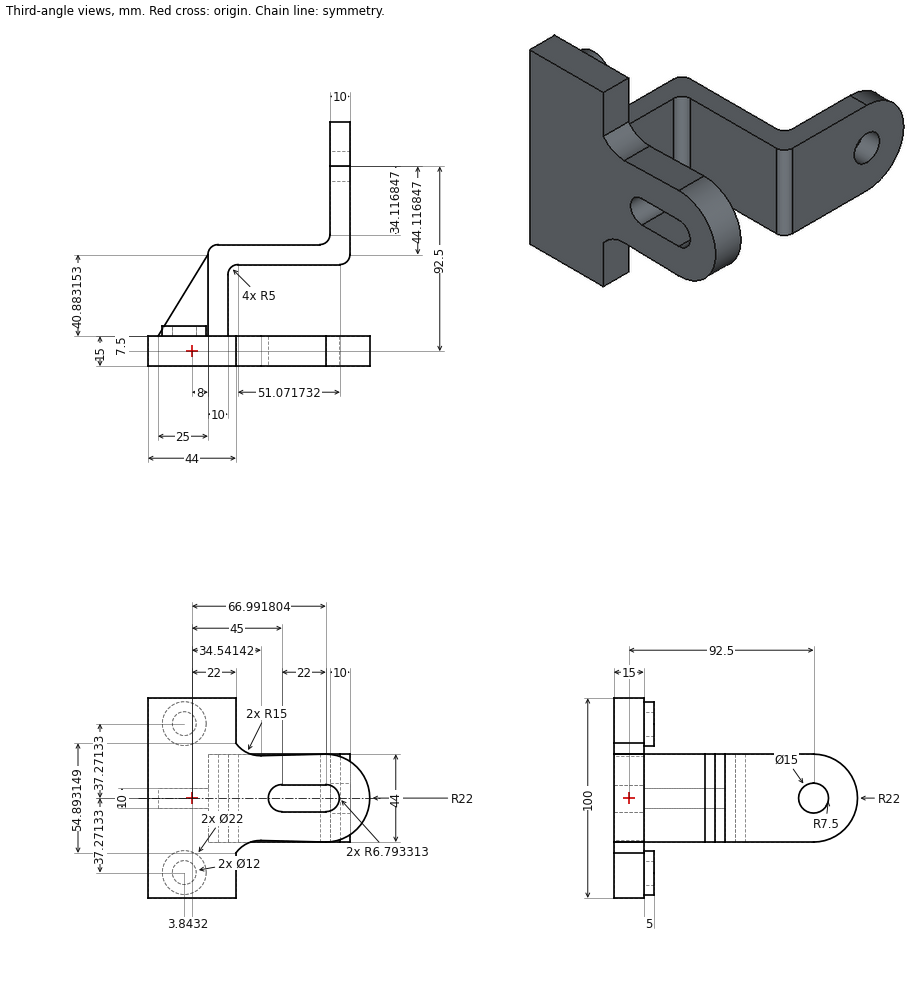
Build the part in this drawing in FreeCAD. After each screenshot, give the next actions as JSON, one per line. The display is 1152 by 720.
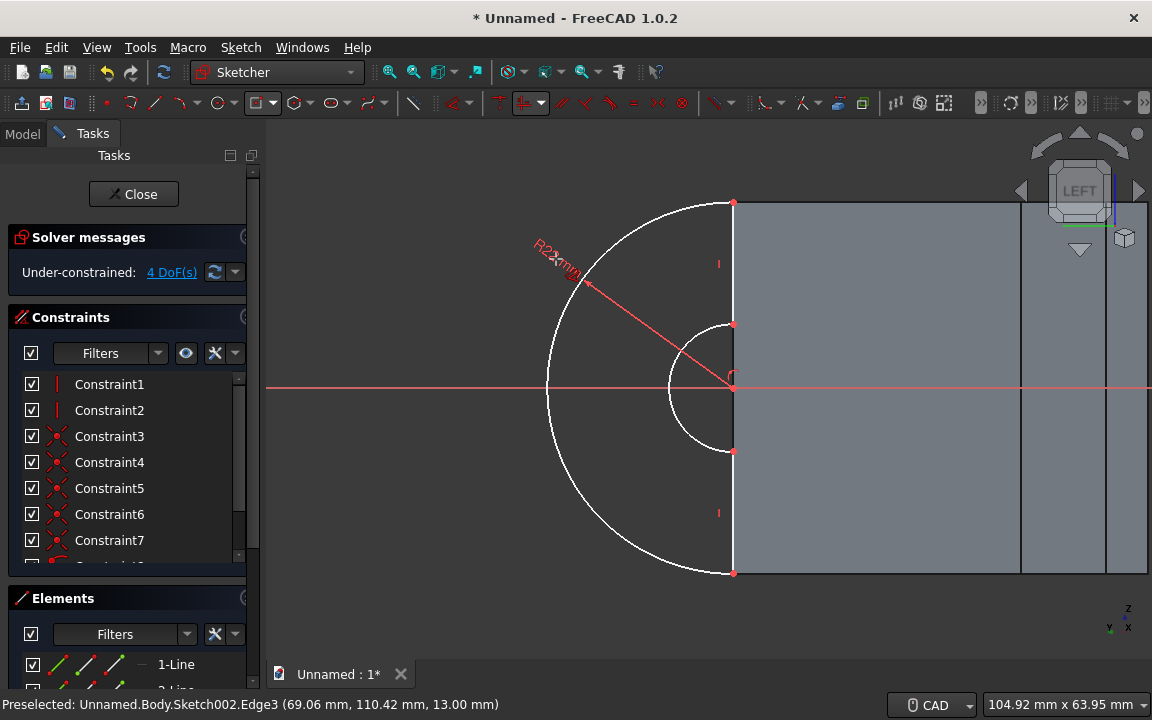
{"action": "left_click", "coordinate": [681, 351]}
{"action": "left_click", "coordinate": [655, 332]}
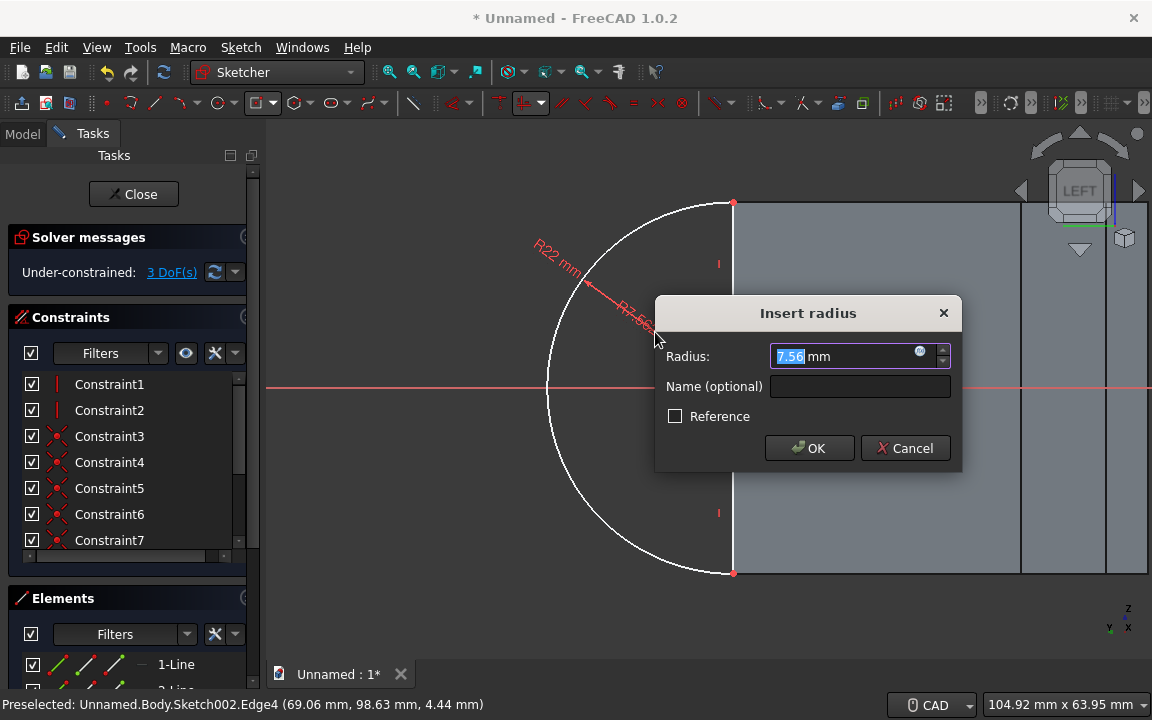
{"action": "type", "text": "7.5"}
{"action": "key", "text": "Return"}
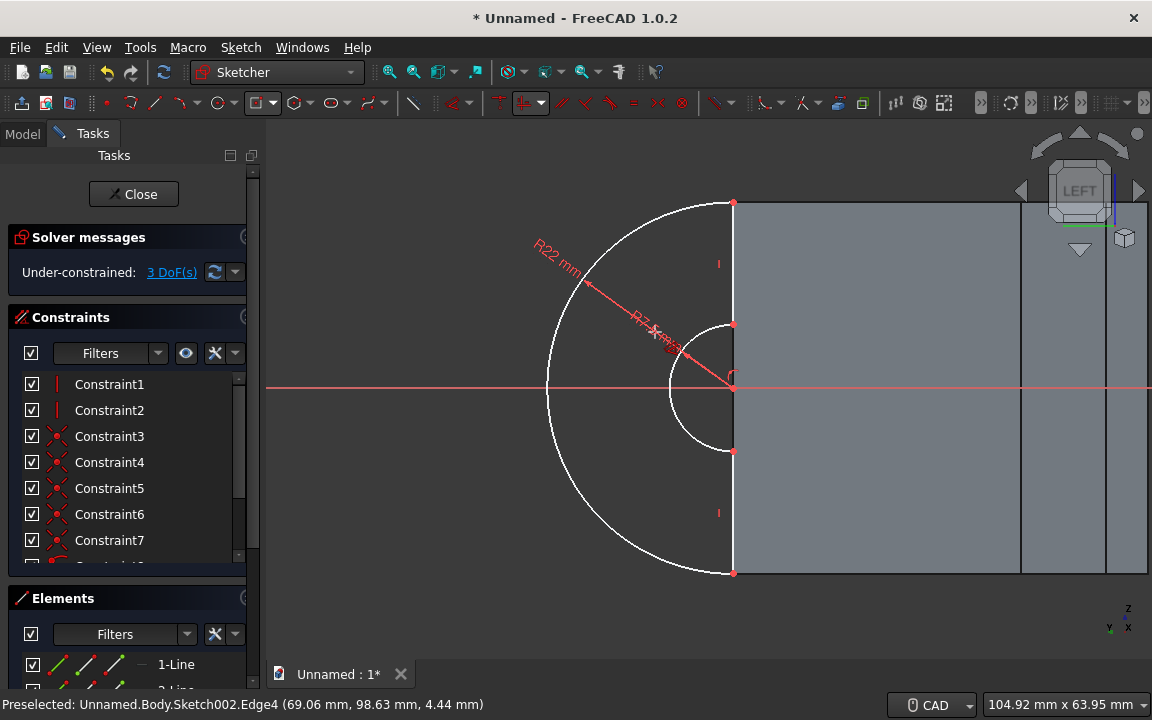
{"action": "left_click", "coordinate": [733, 325]}
{"action": "left_click", "coordinate": [860, 291]}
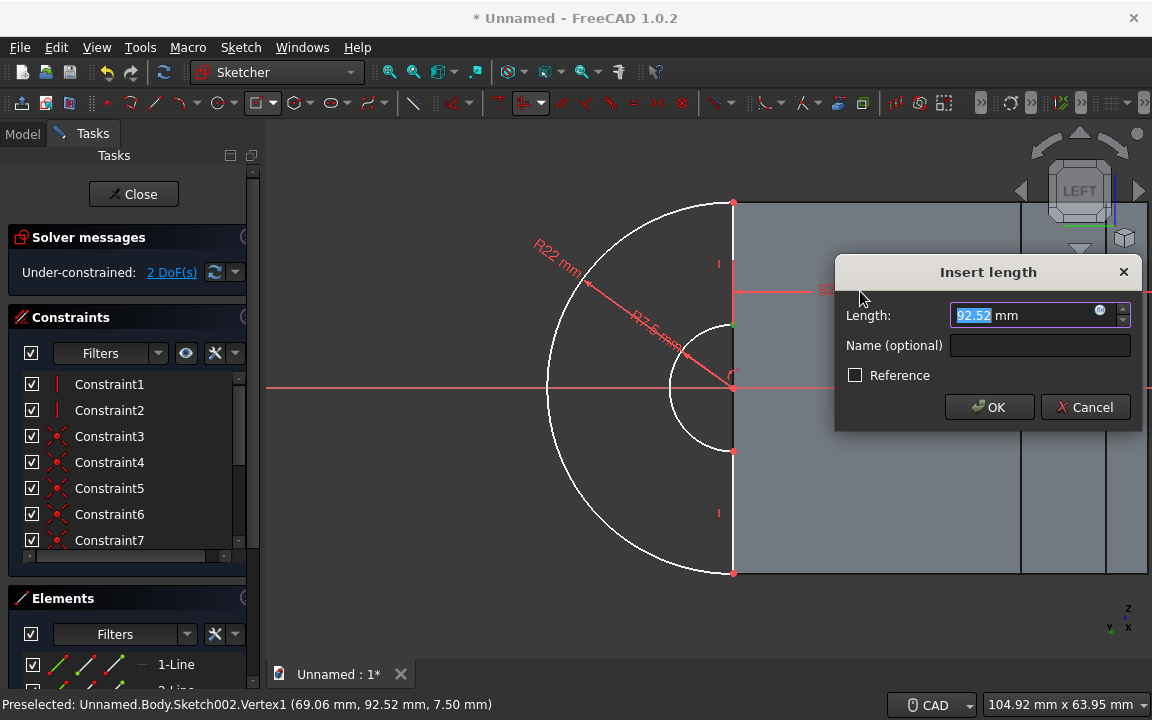
{"action": "type", "text": "92.5"}
{"action": "key", "text": "Return"}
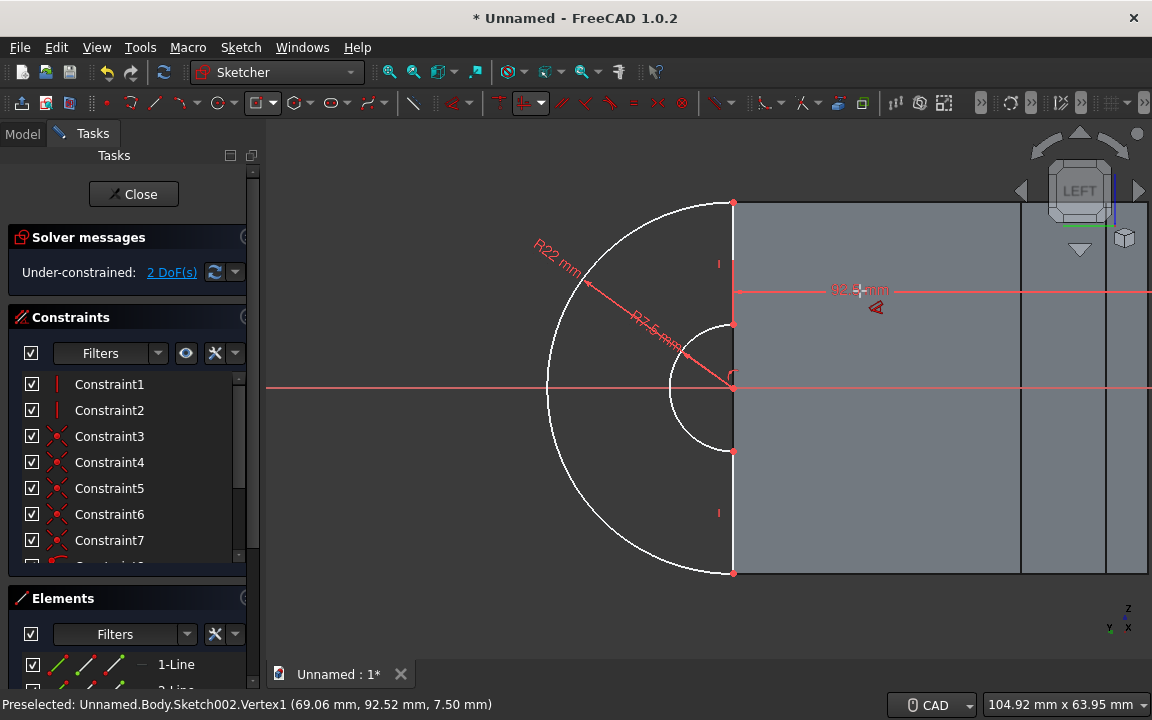
{"action": "left_click", "coordinate": [733, 574]}
{"action": "left_click", "coordinate": [860, 608]}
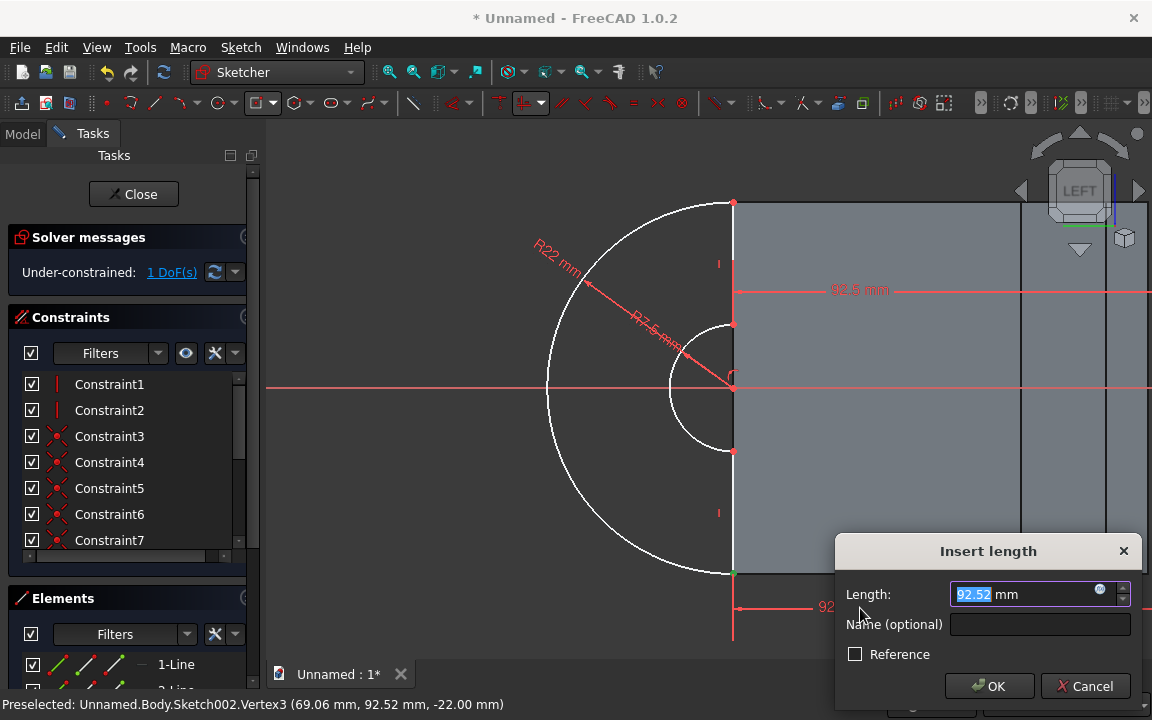
{"action": "type", "text": "92.5"}
{"action": "key", "text": "Return"}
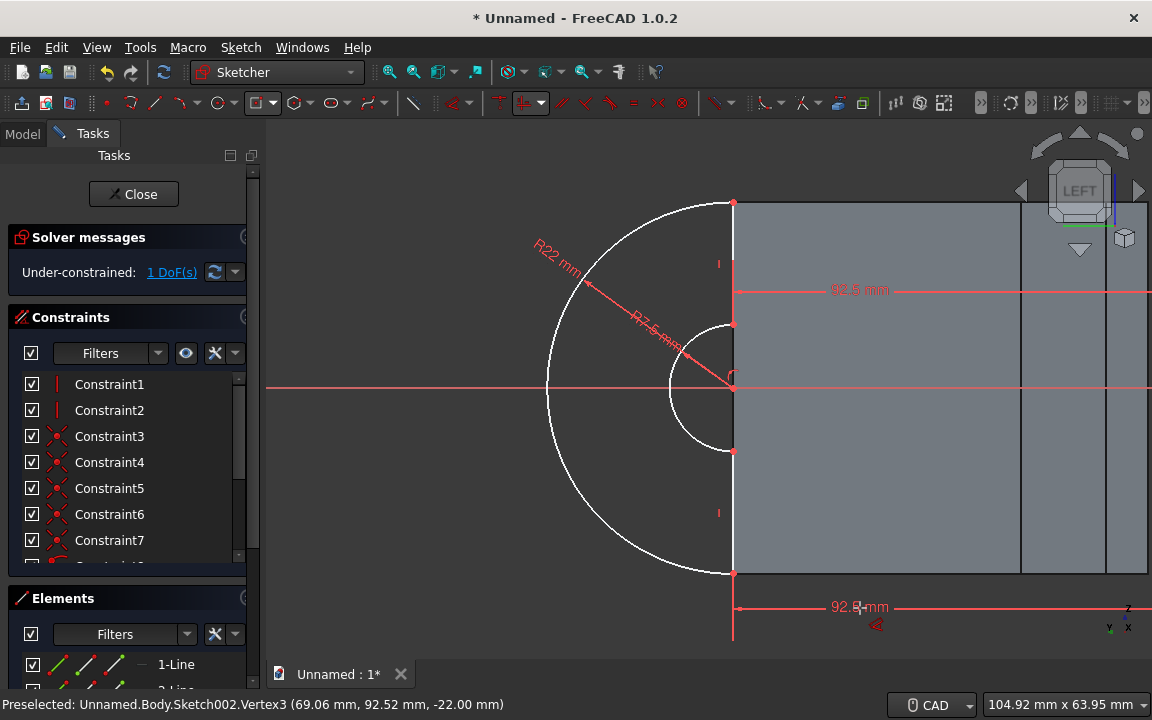
{"action": "left_click", "coordinate": [733, 388]}
{"action": "left_click", "coordinate": [860, 422]}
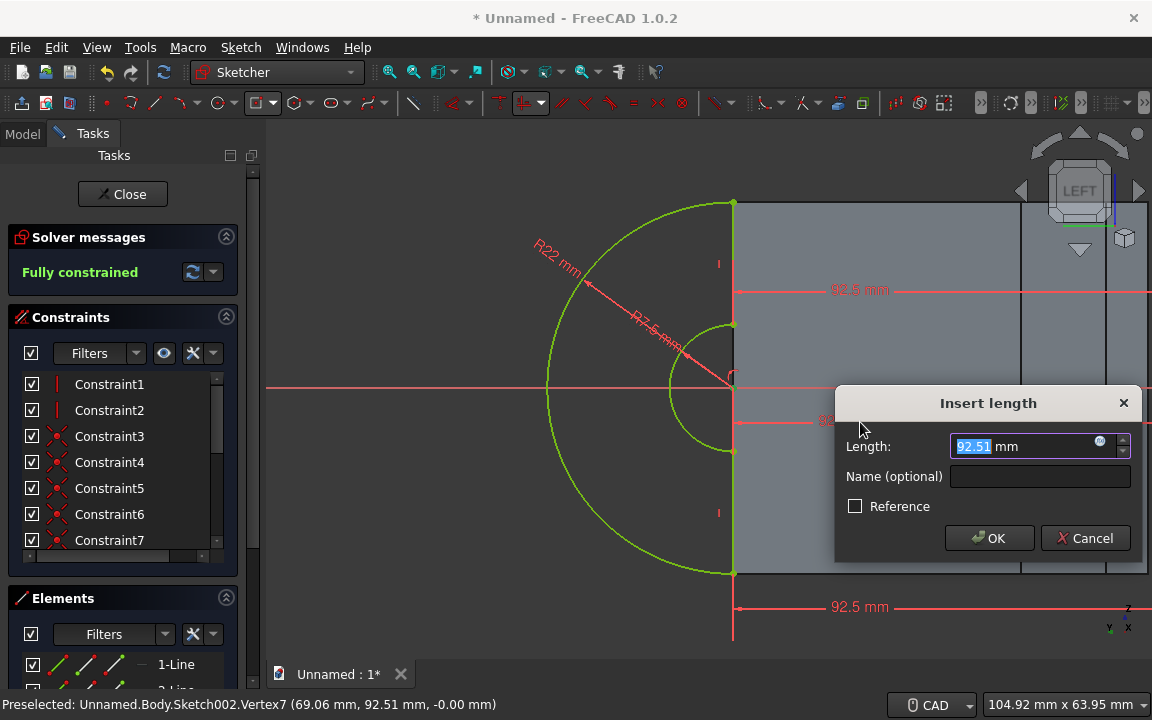
{"action": "type", "text": "92.5"}
{"action": "key", "text": "Return"}
{"action": "key", "text": "Escape"}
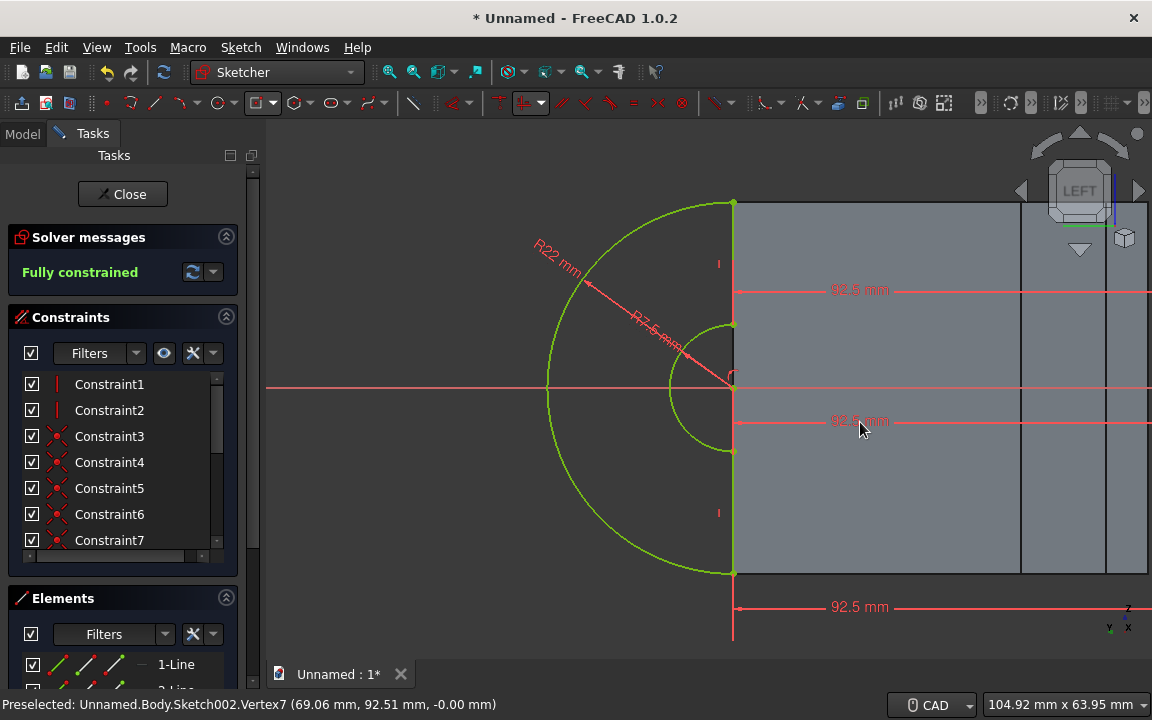
{"action": "left_click", "coordinate": [123, 194]}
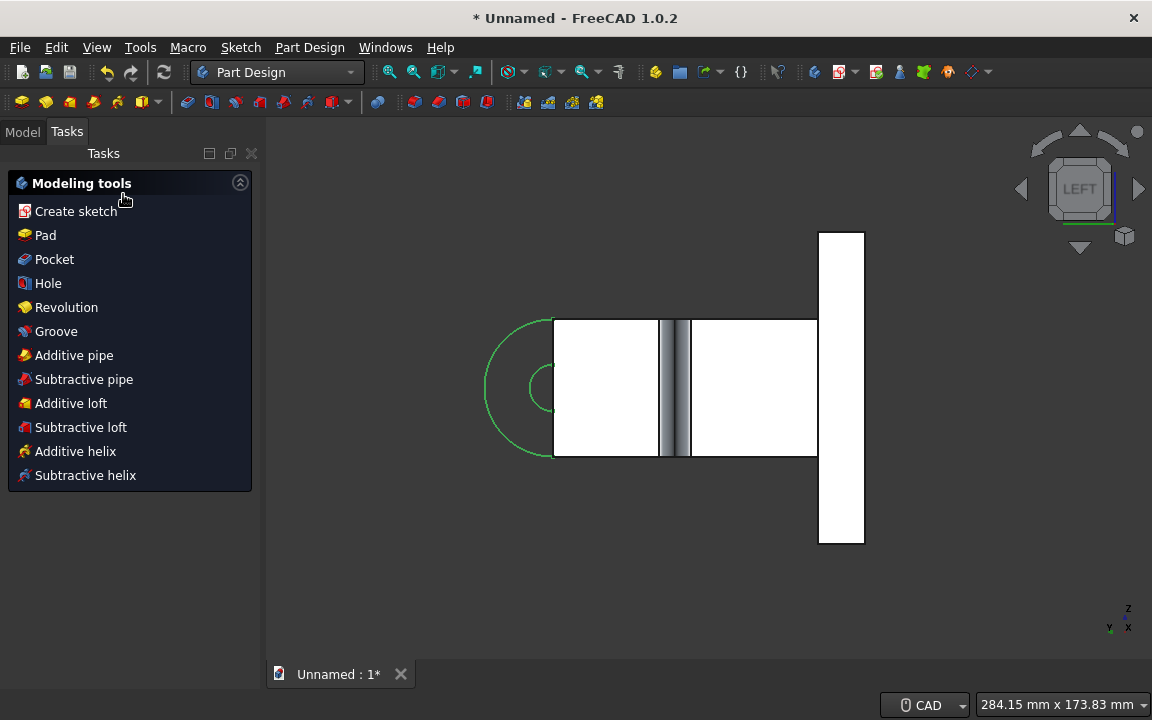
{"action": "left_click", "coordinate": [22, 102]}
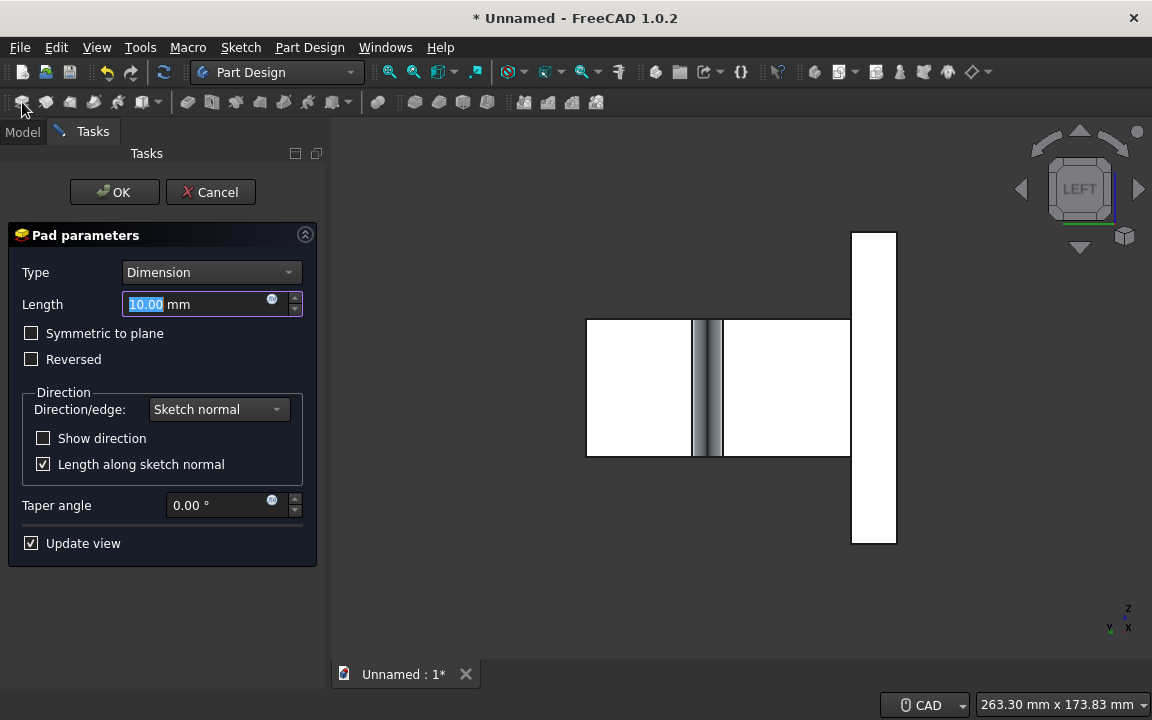
{"action": "type", "text": "10"}
{"action": "key", "text": "Tab"}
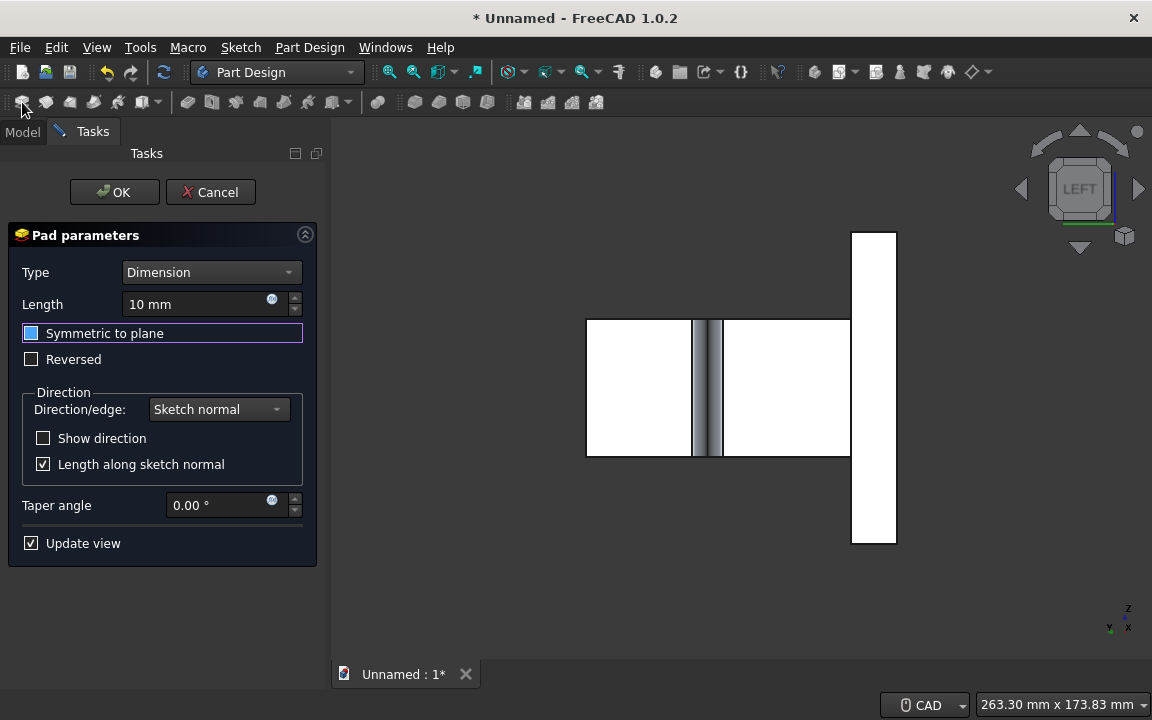
{"action": "left_click", "coordinate": [30, 359]}